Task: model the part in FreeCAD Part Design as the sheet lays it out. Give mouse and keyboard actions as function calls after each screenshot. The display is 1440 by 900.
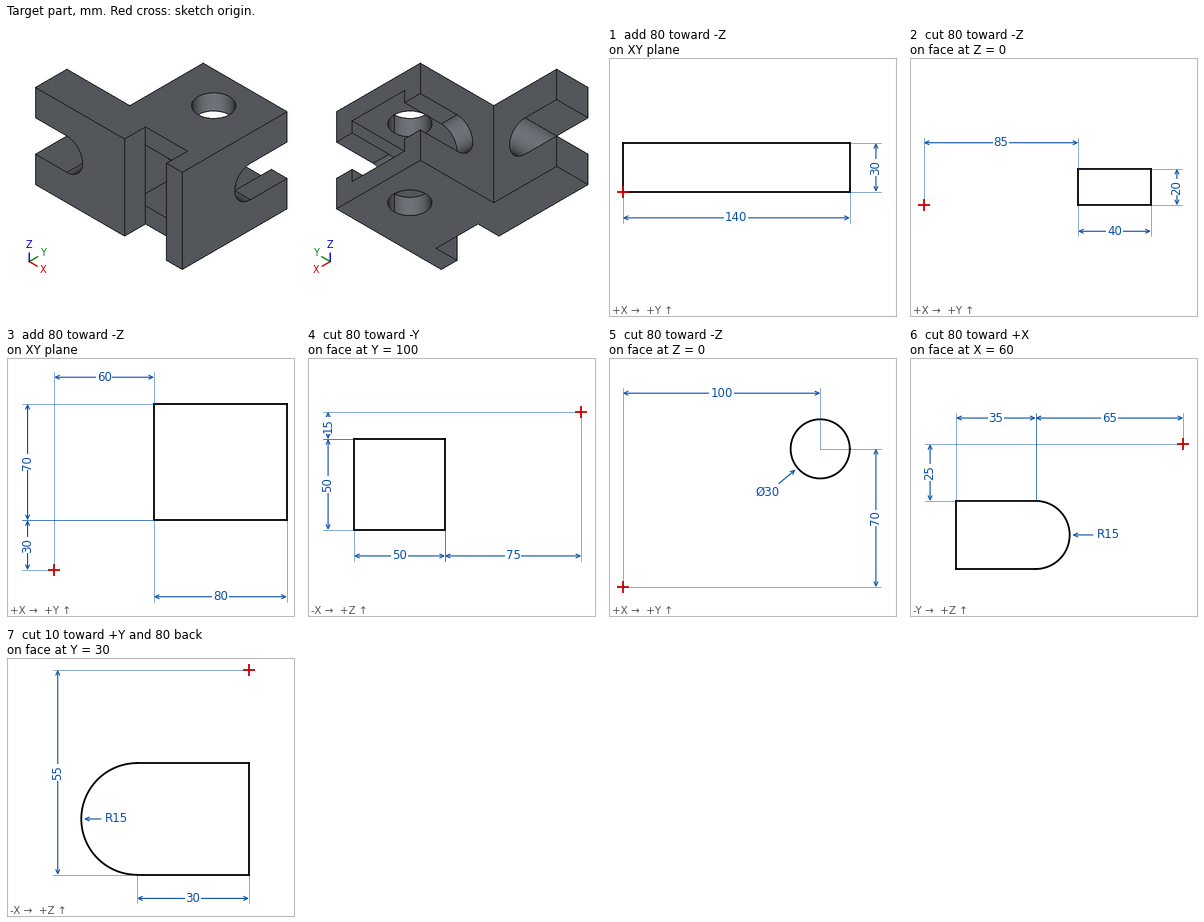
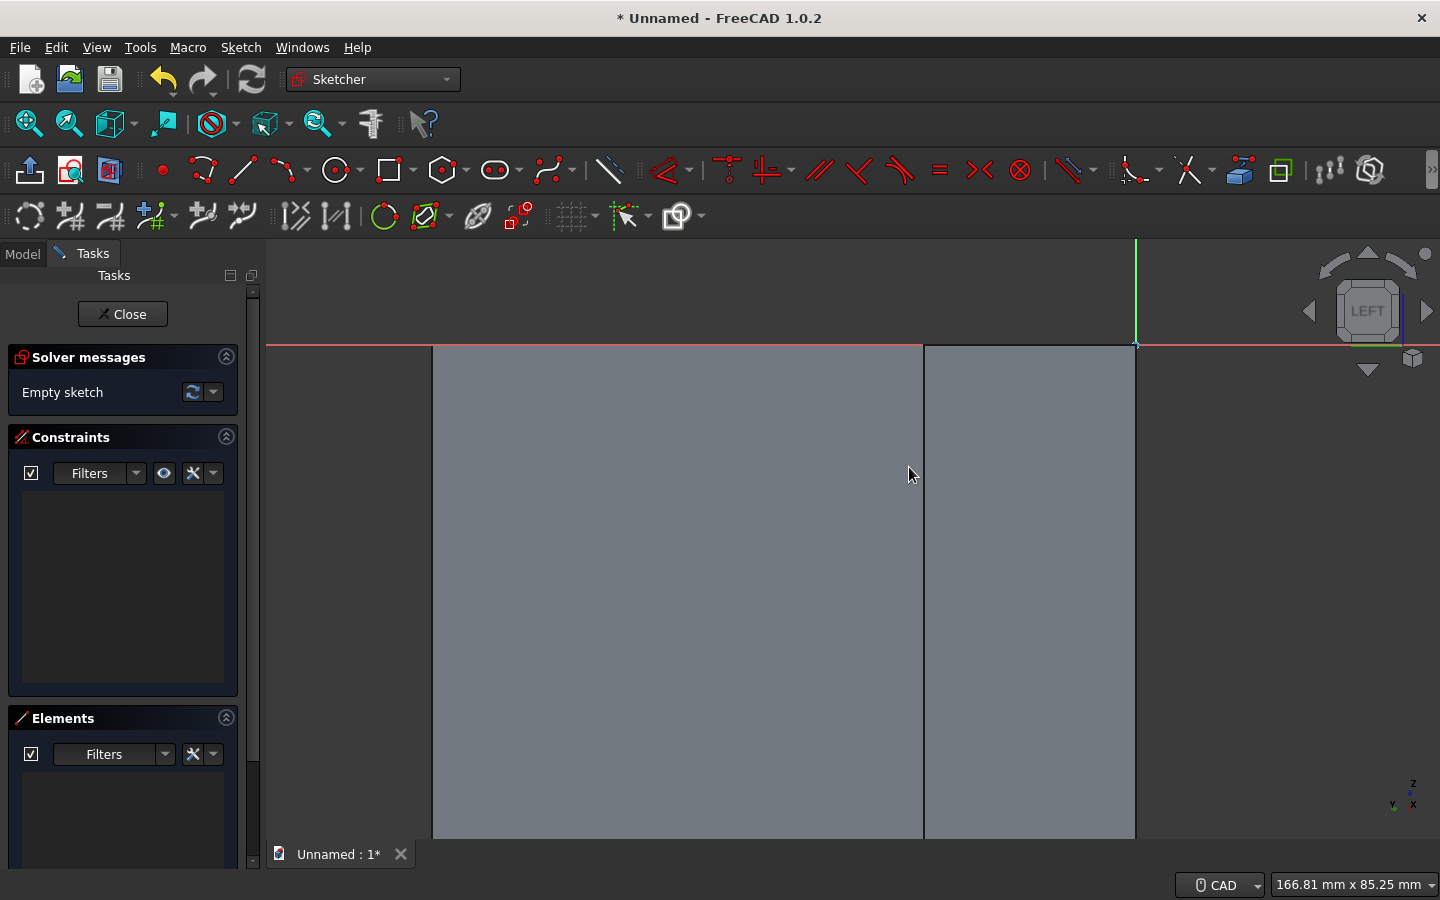
key(g)
key(m)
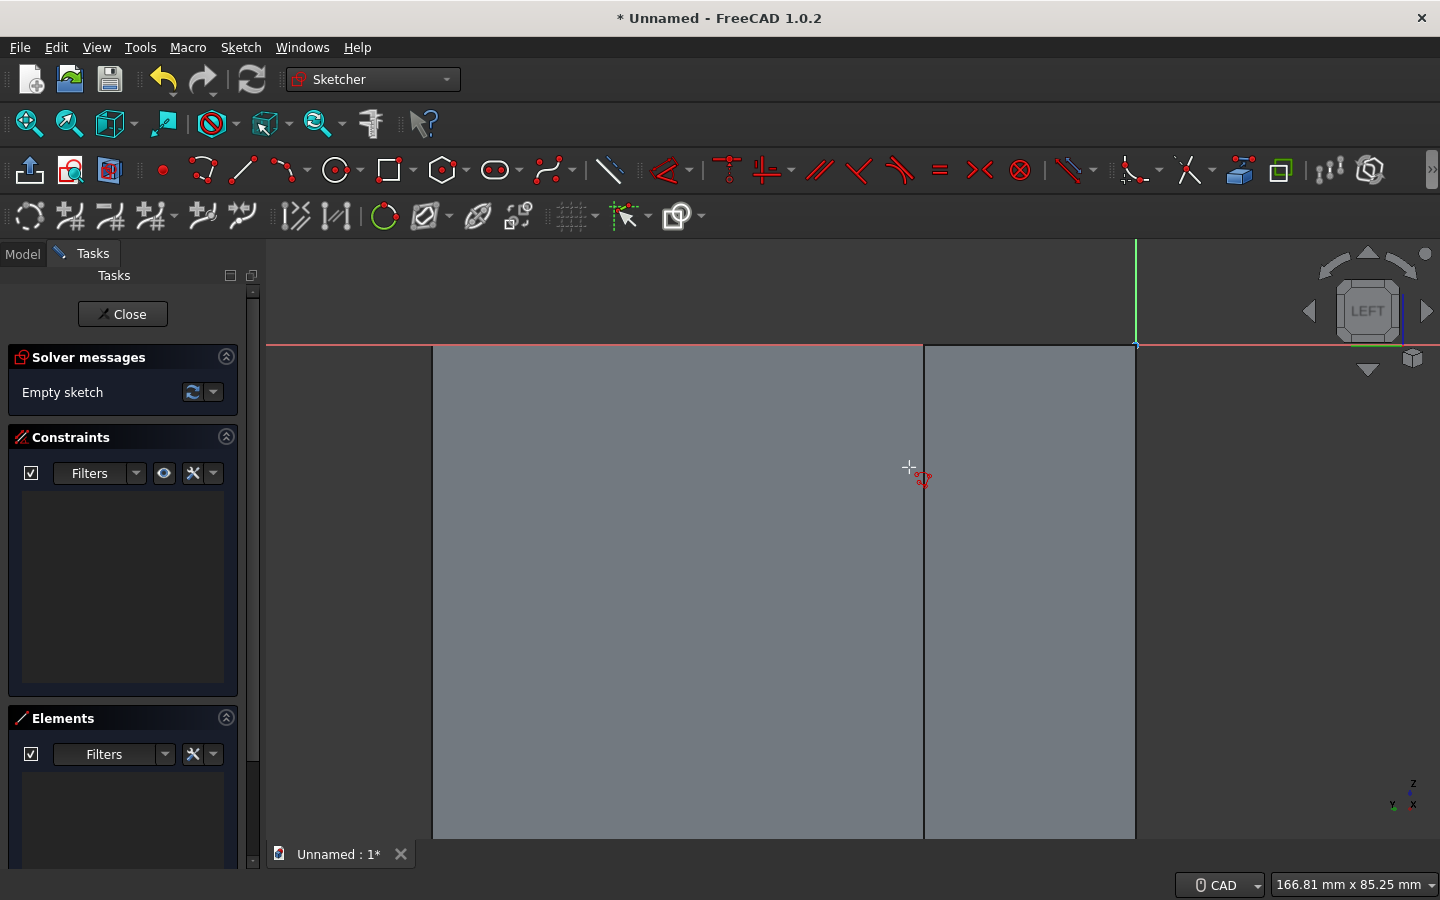
click(678, 521)
click(432, 521)
click(432, 732)
click(678, 732)
right_click(678, 732)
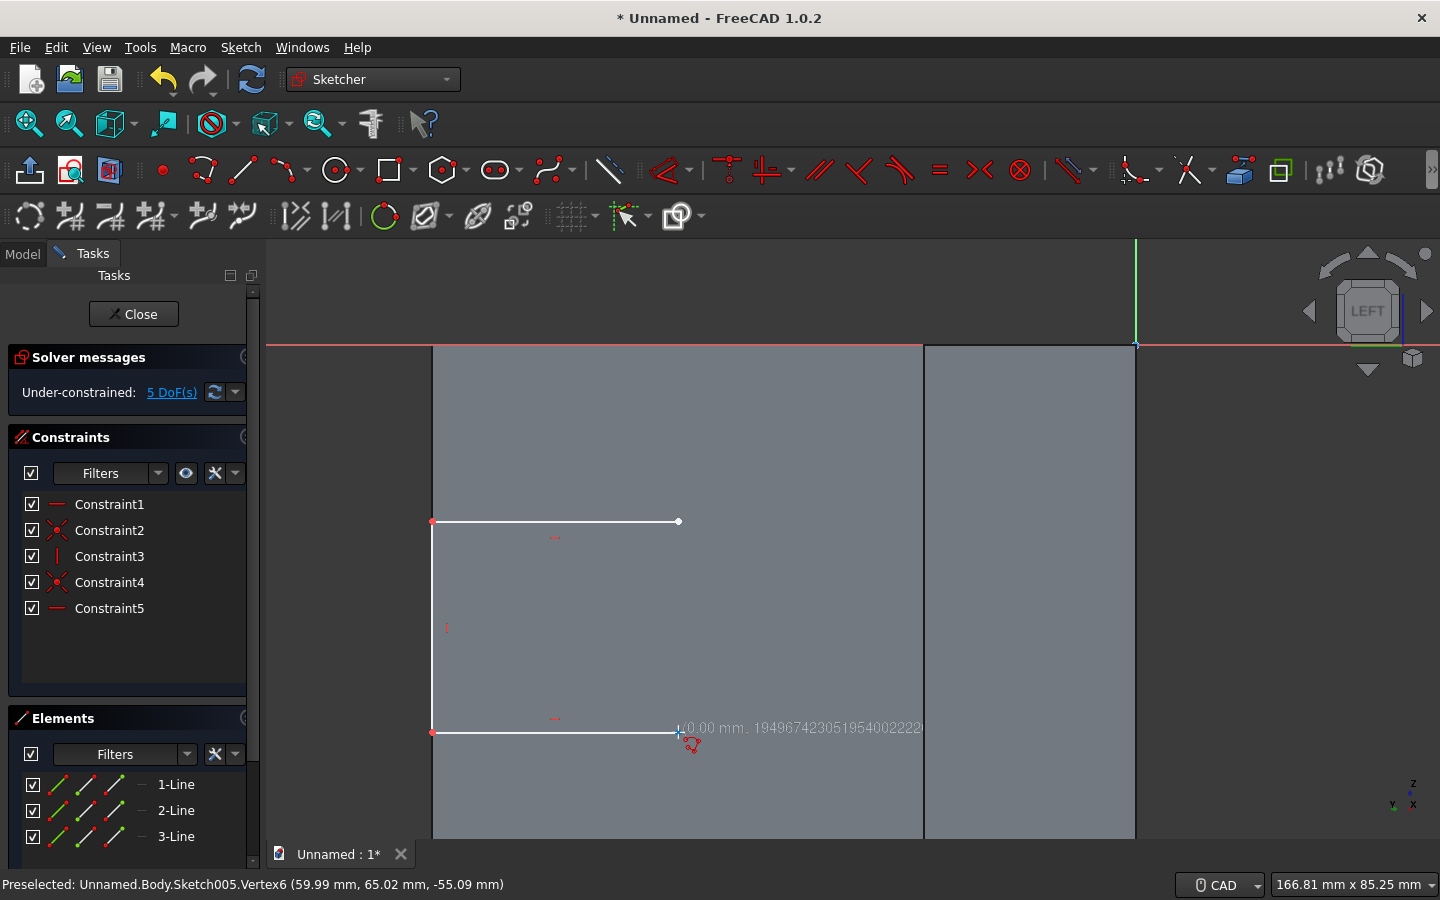
key(g)
key(3)
key(a)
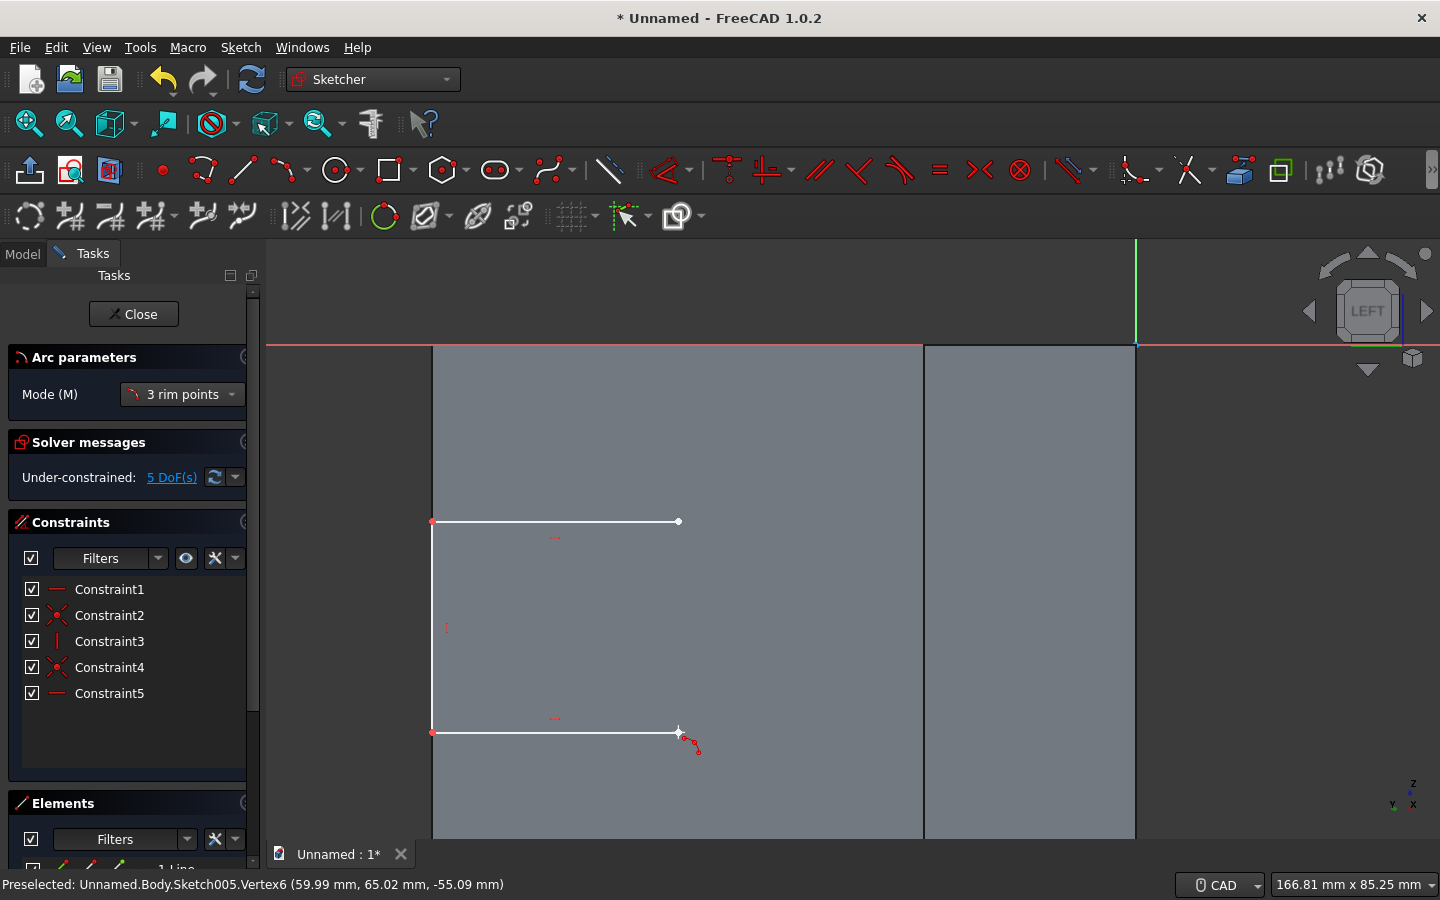
click(678, 733)
click(678, 522)
click(784, 627)
key(Escape)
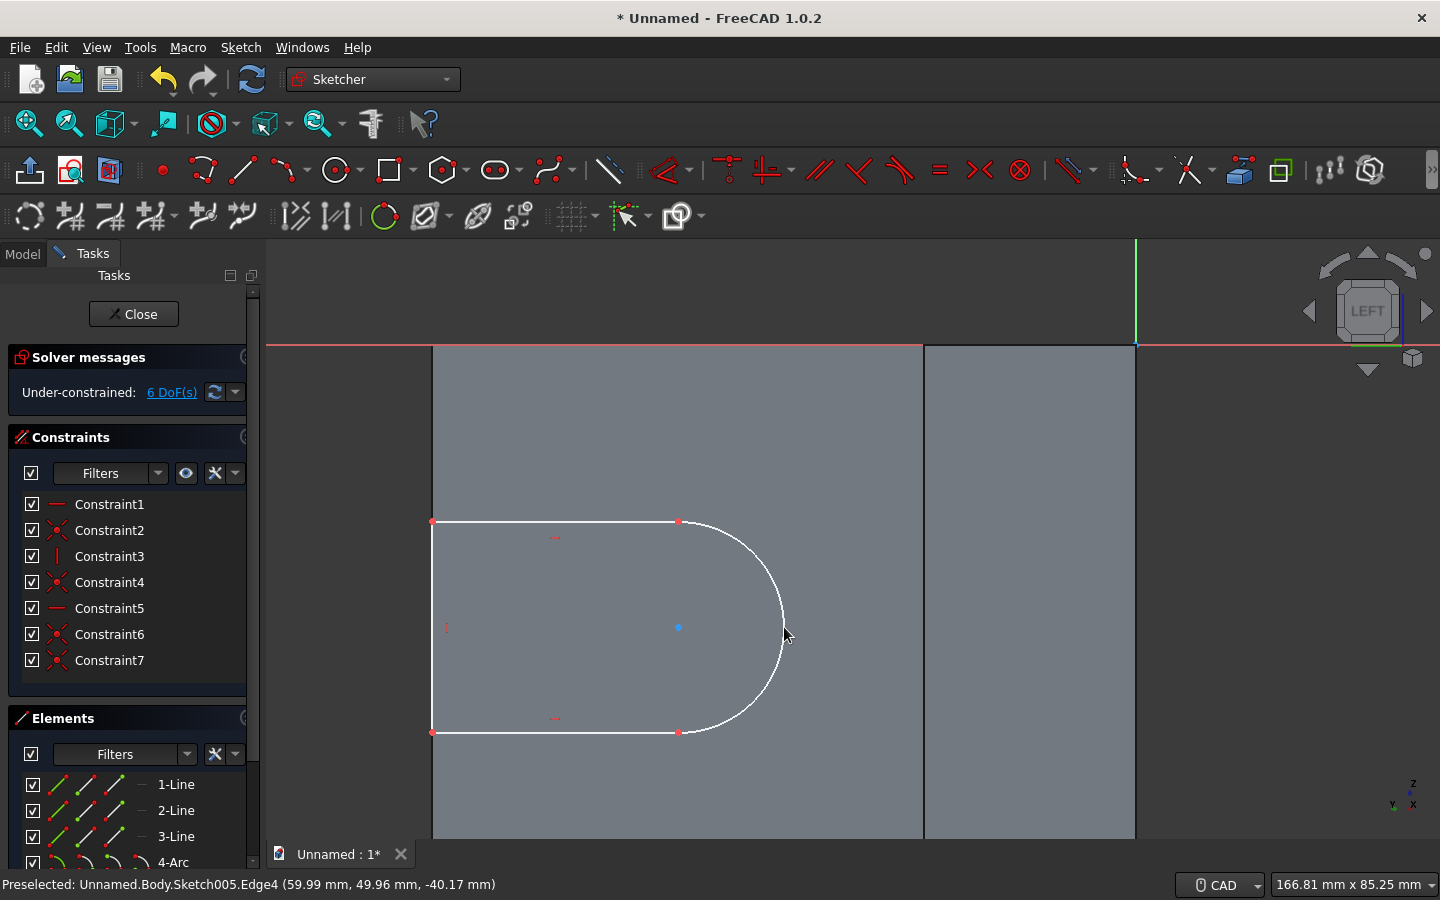
click(604, 522)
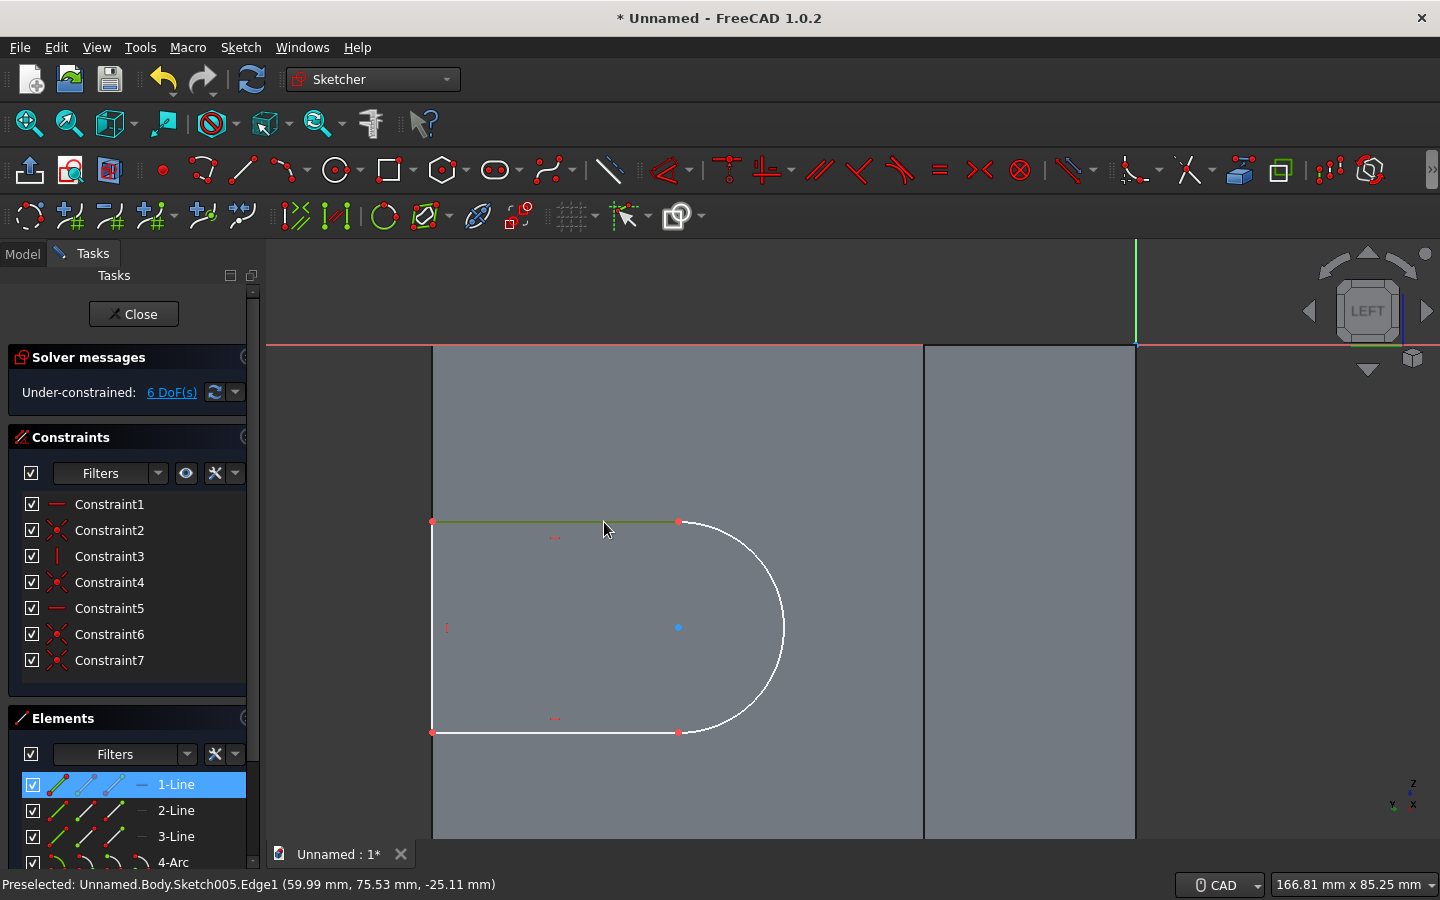
click(764, 690)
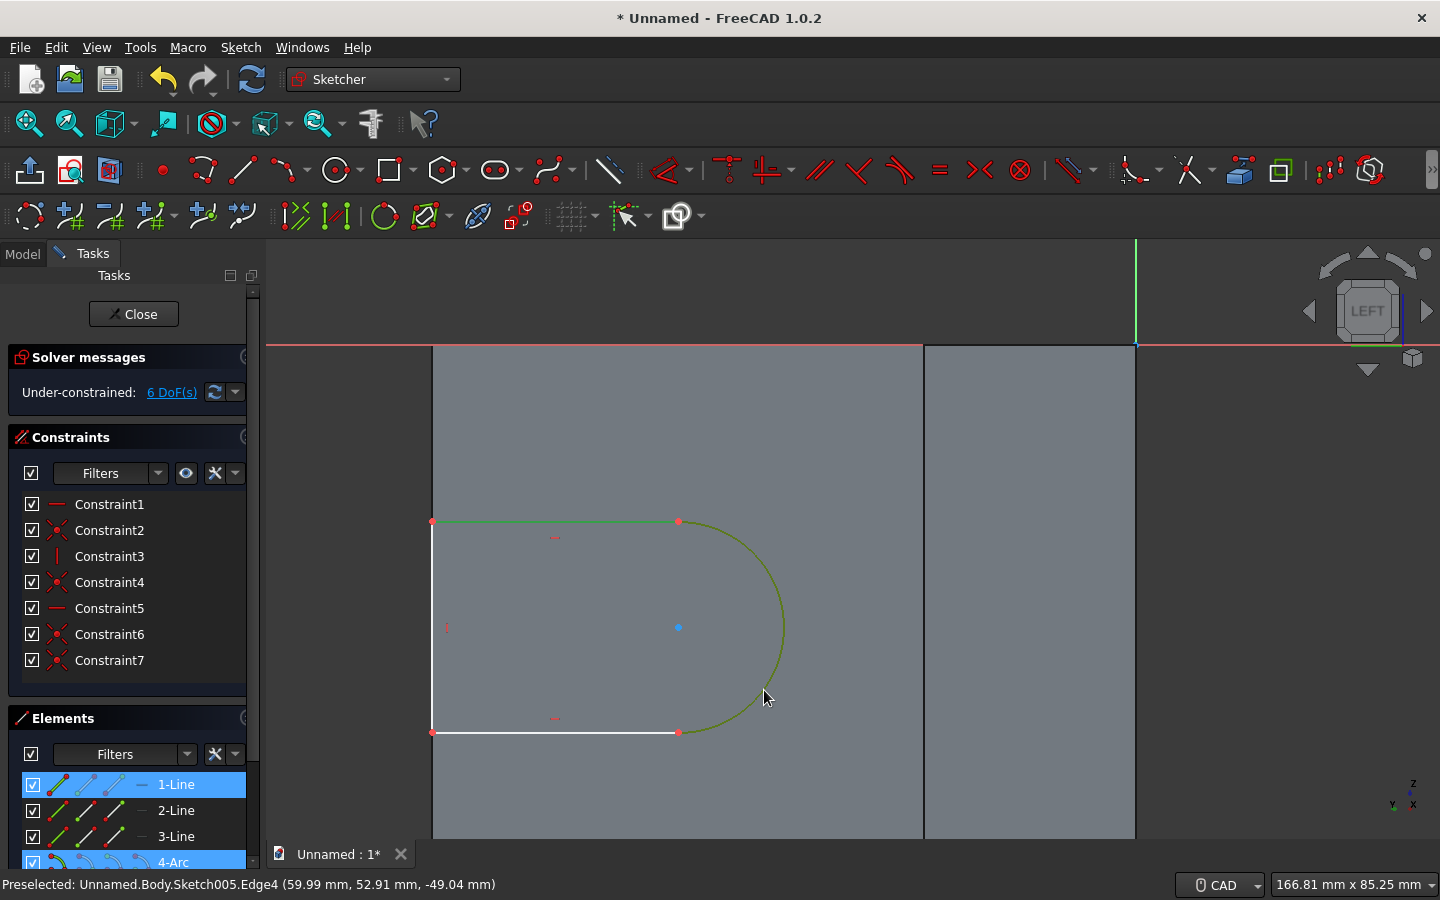
click(900, 170)